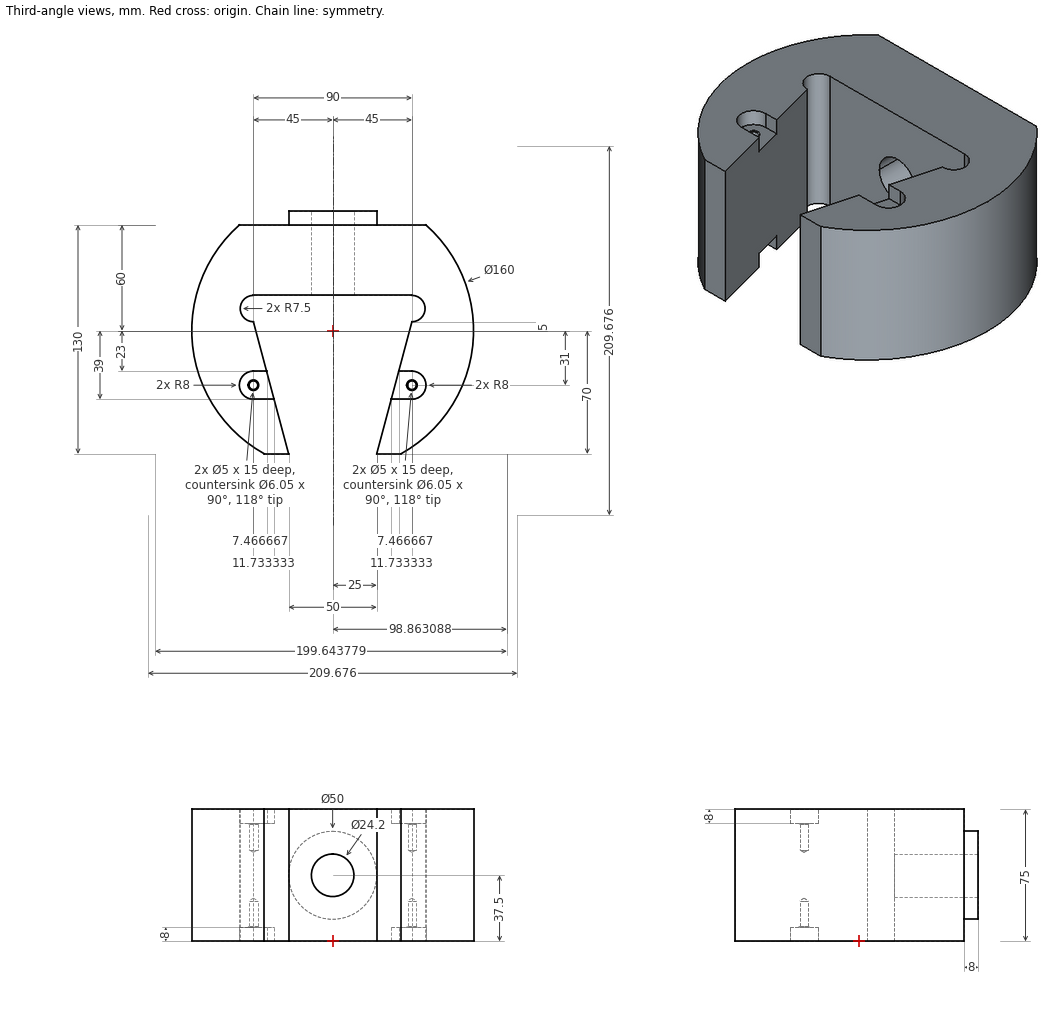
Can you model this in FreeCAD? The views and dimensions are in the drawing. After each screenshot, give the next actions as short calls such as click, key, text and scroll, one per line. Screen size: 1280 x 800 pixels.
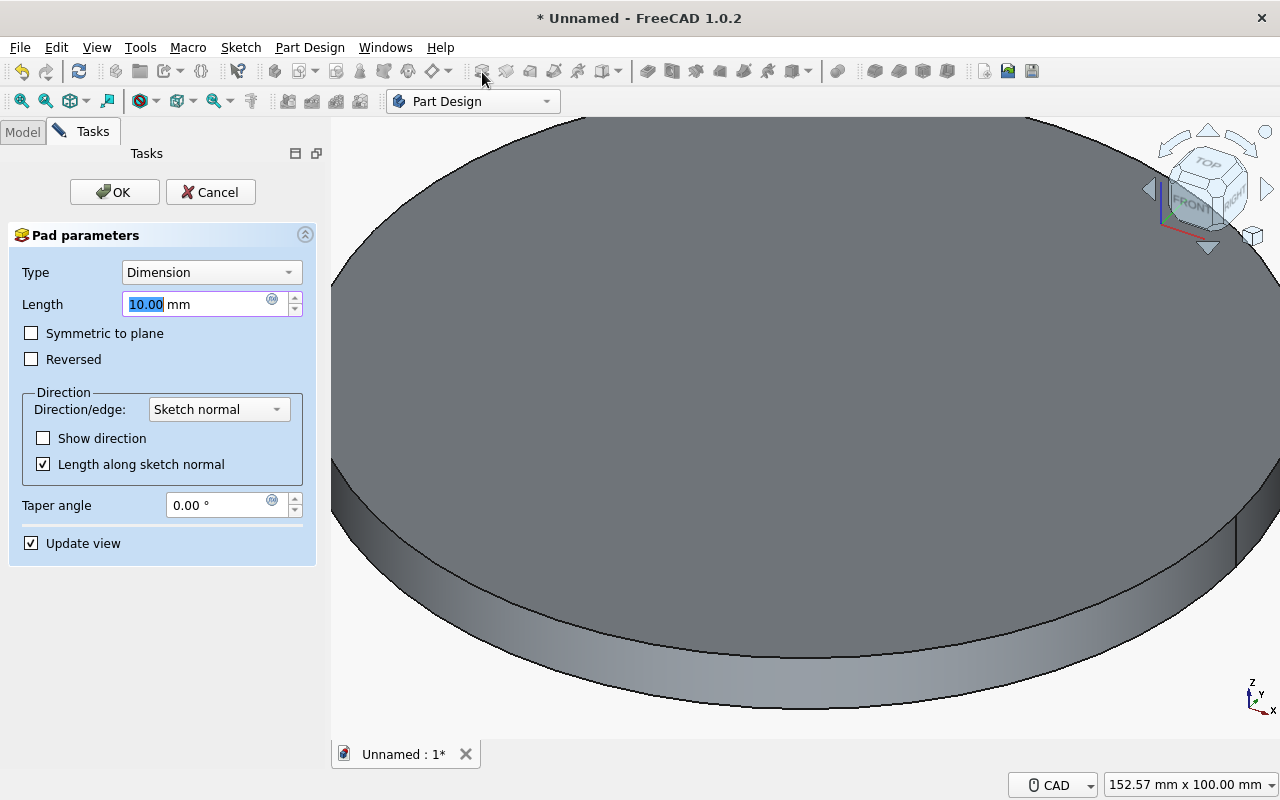
text(75)
key(Tab)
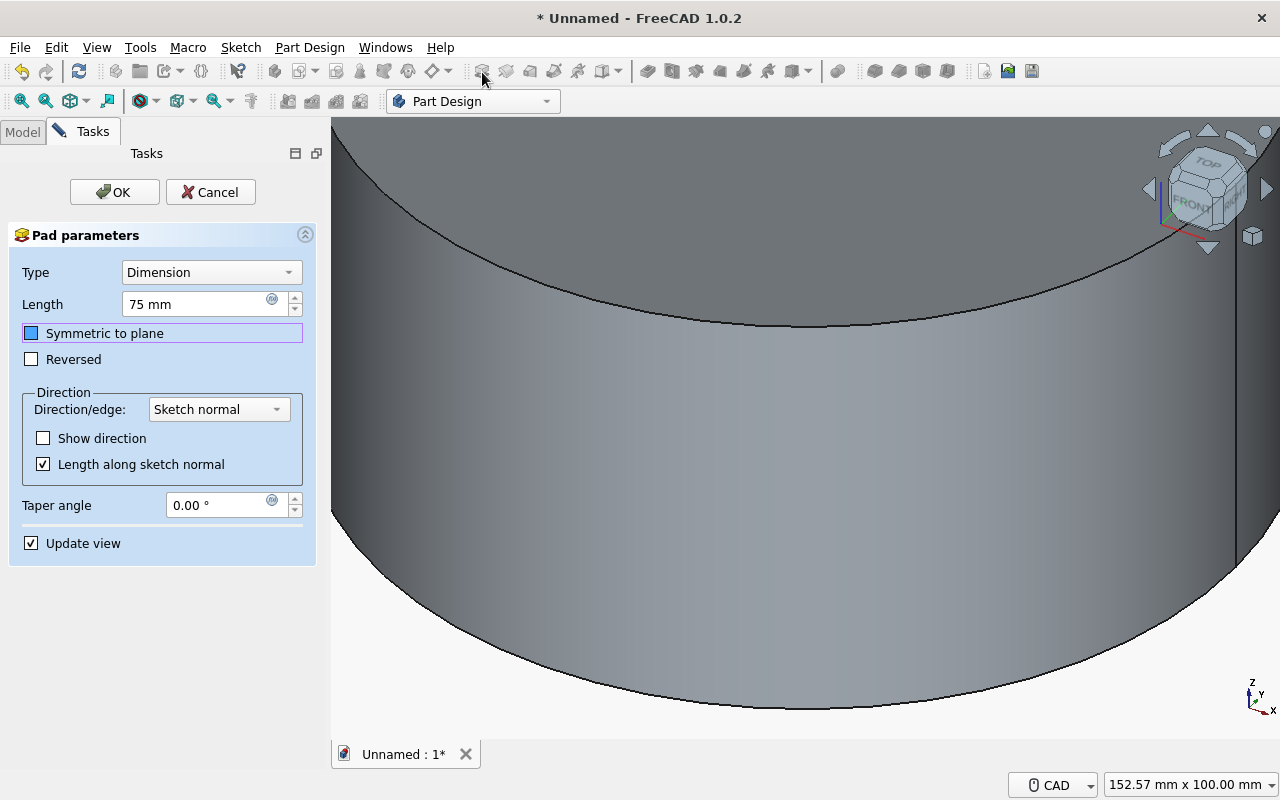
click(115, 192)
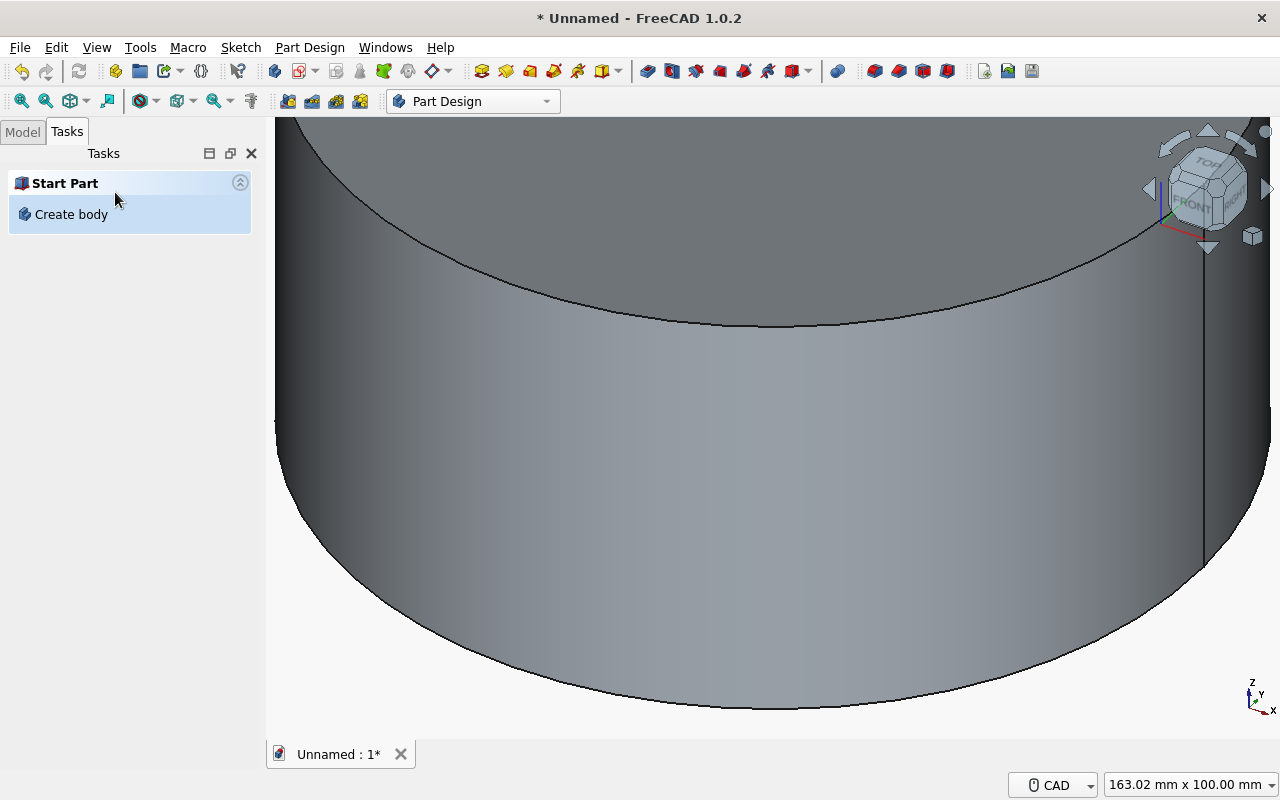
key(v)
key(f)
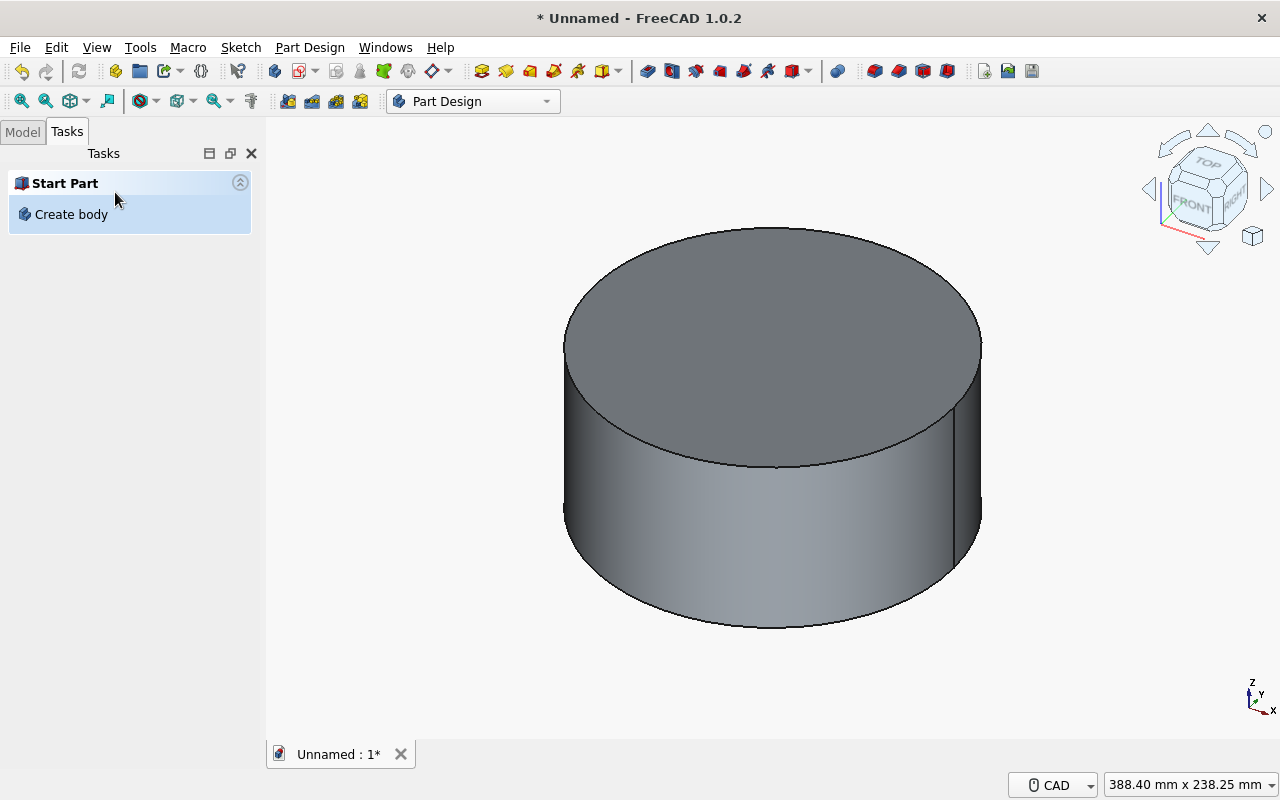
click(300, 72)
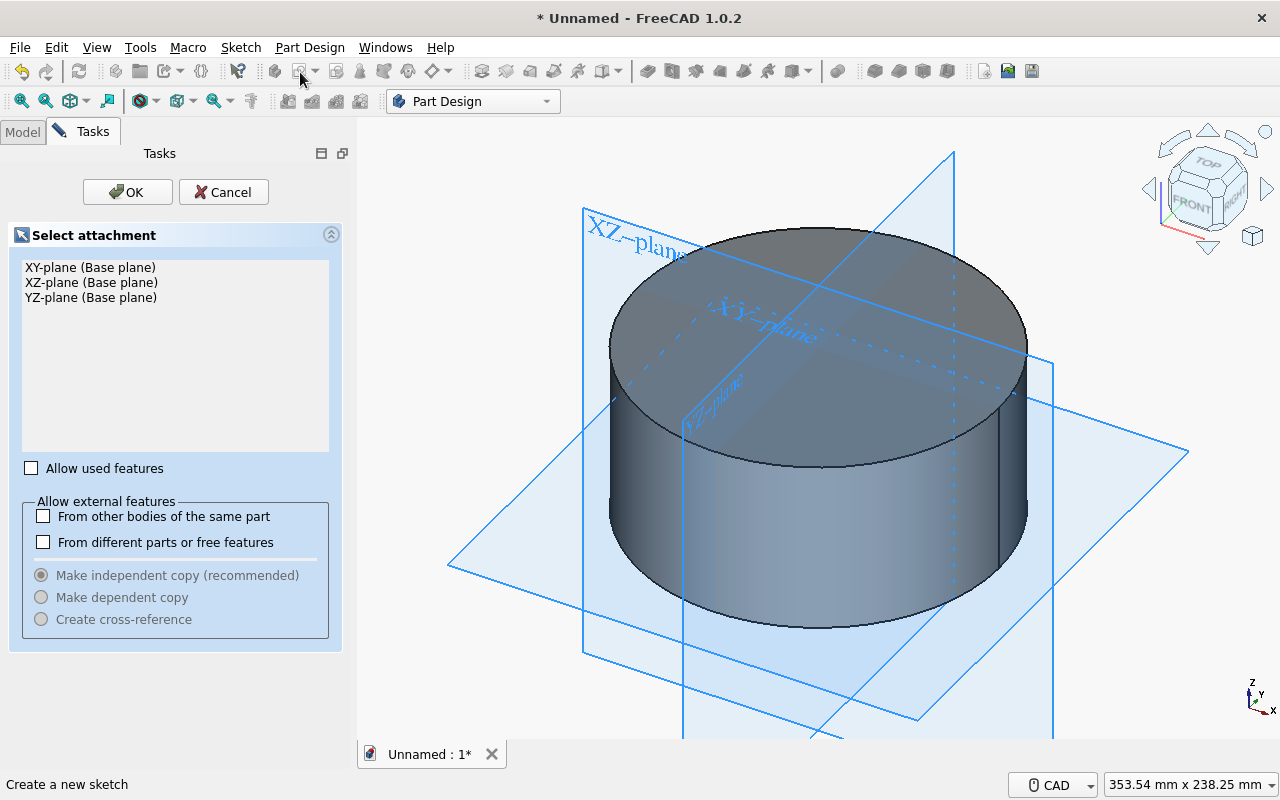
click(82, 268)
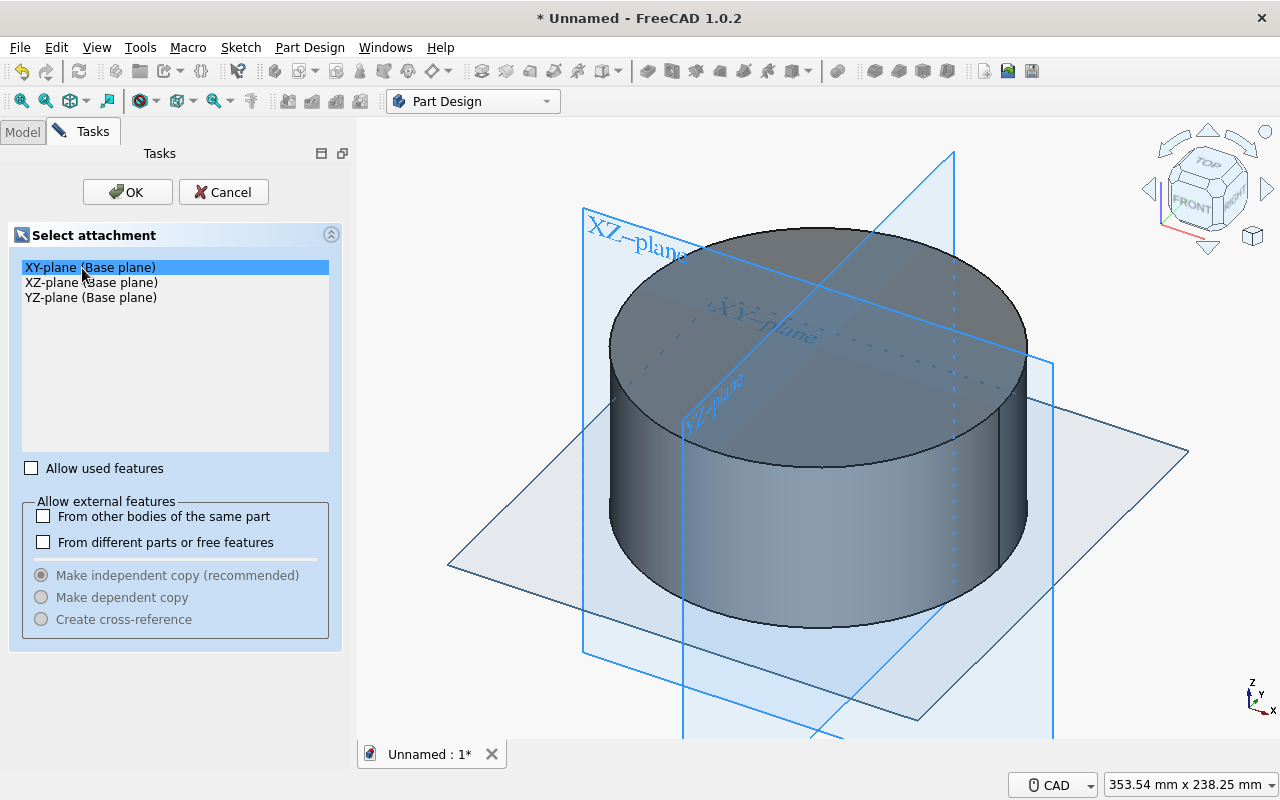
click(128, 192)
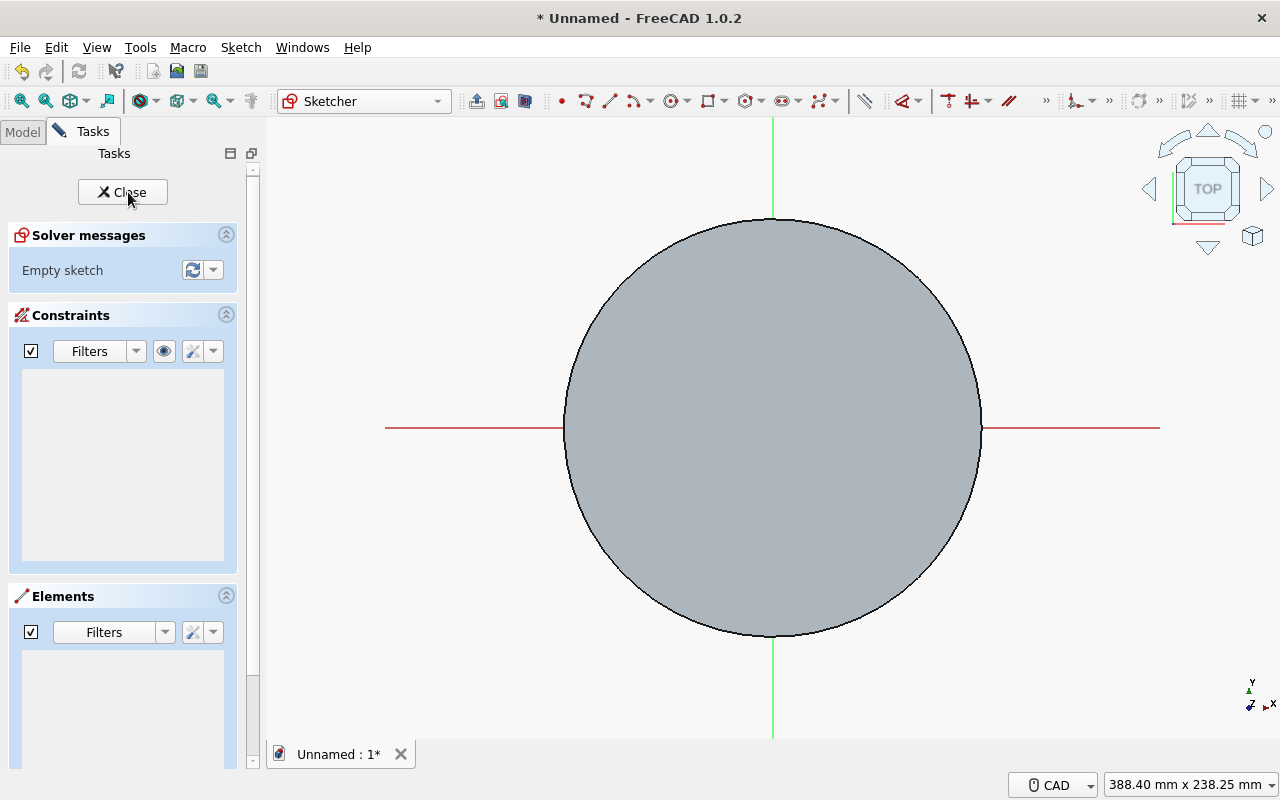
key(q)
key(s)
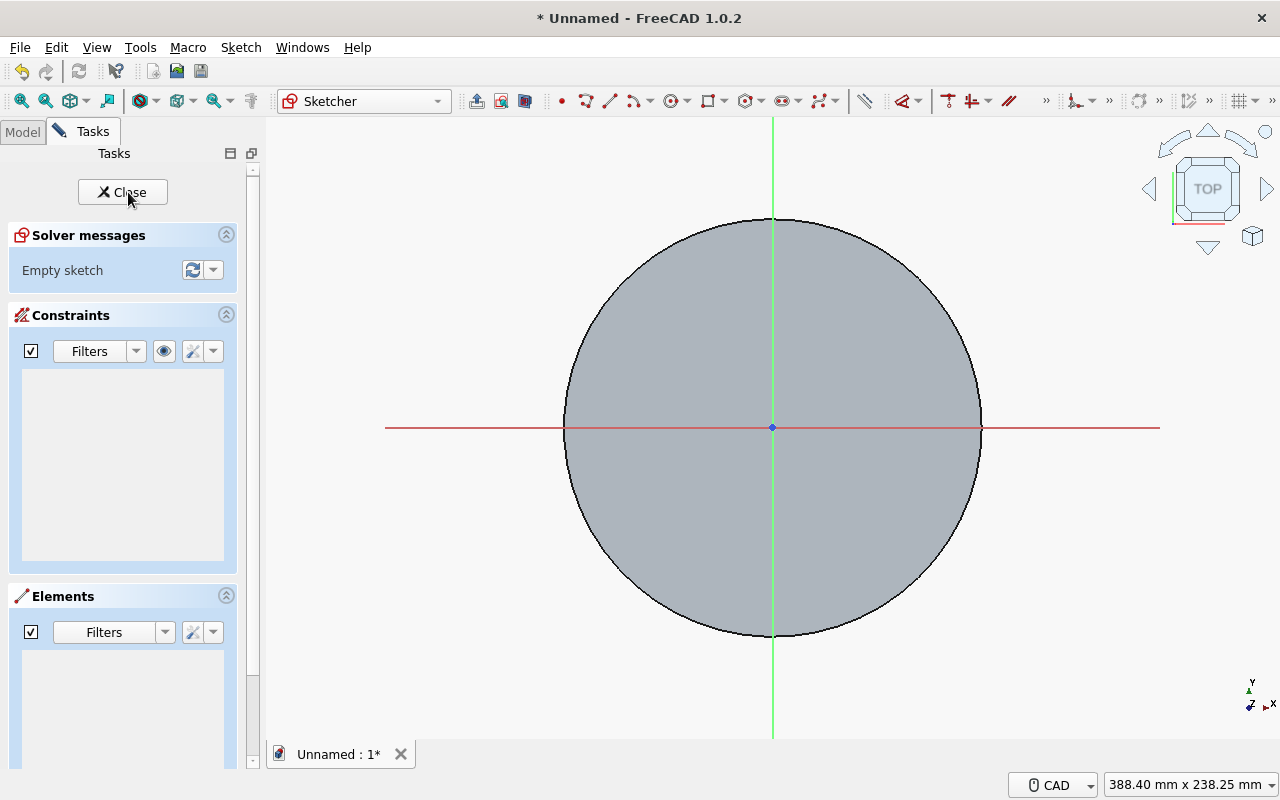
scroll(566, 428, down, 2)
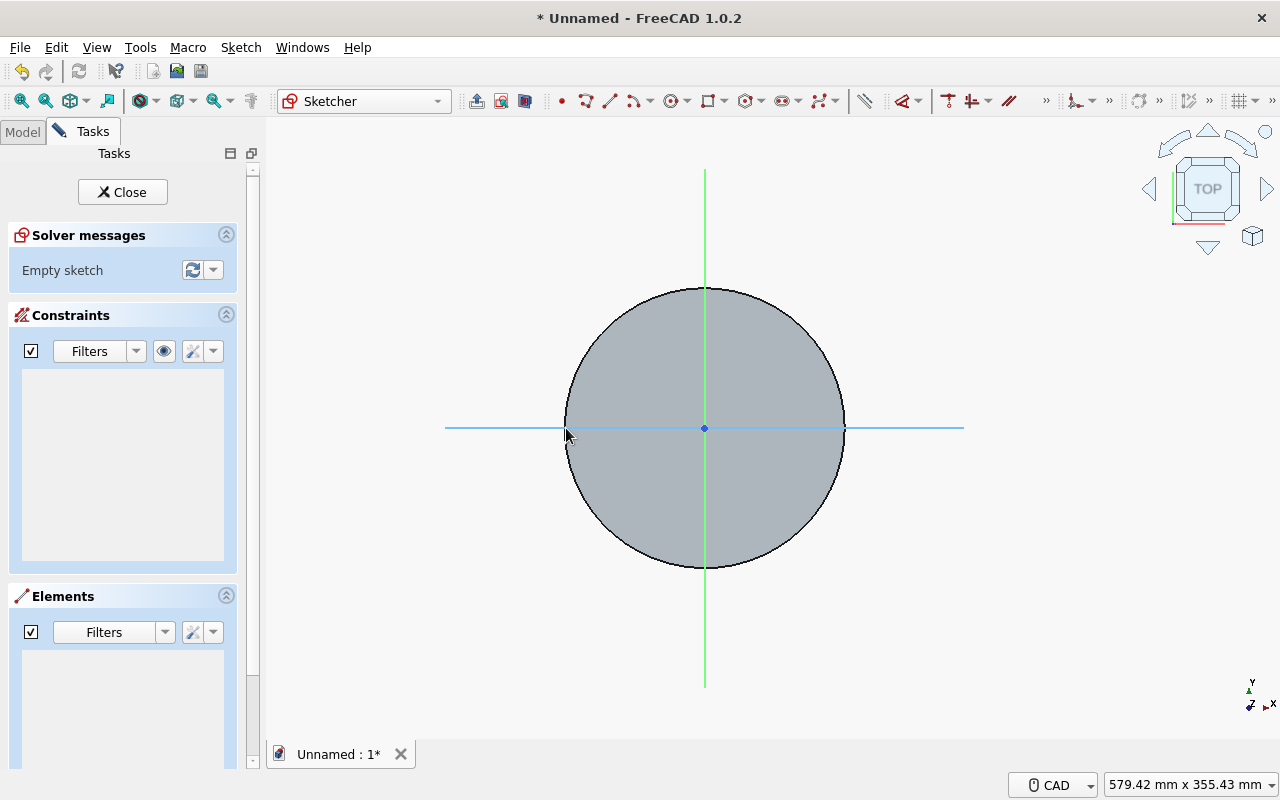
key(g)
key(v)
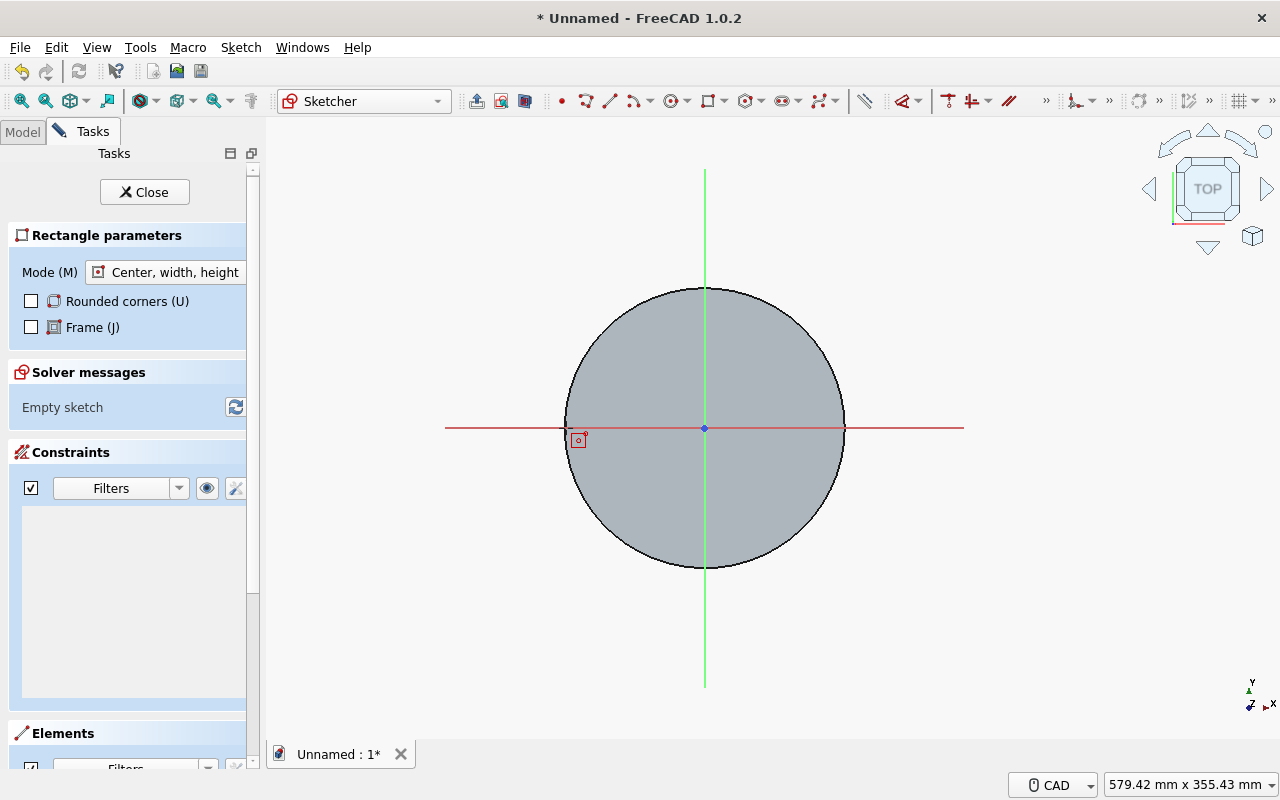
click(705, 428)
move(888, 245)